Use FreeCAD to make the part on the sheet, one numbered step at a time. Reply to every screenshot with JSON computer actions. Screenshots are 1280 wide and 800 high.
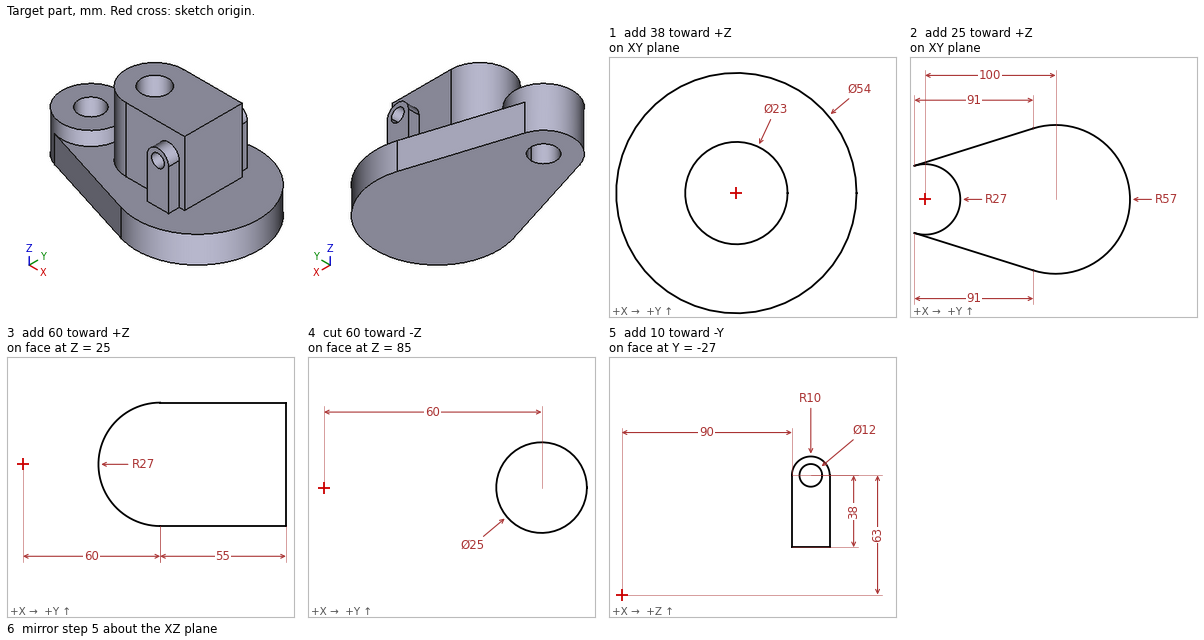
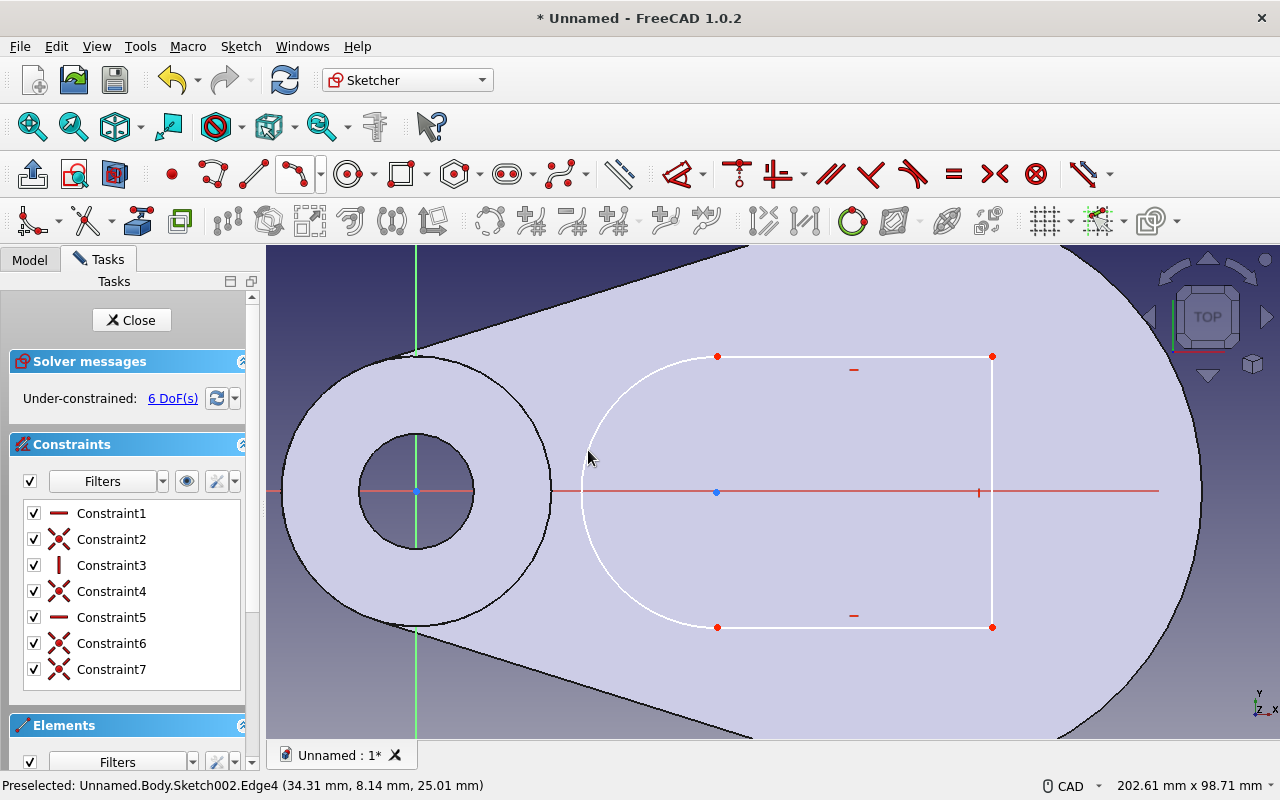
{"action": "left_click", "coordinate": [800, 628]}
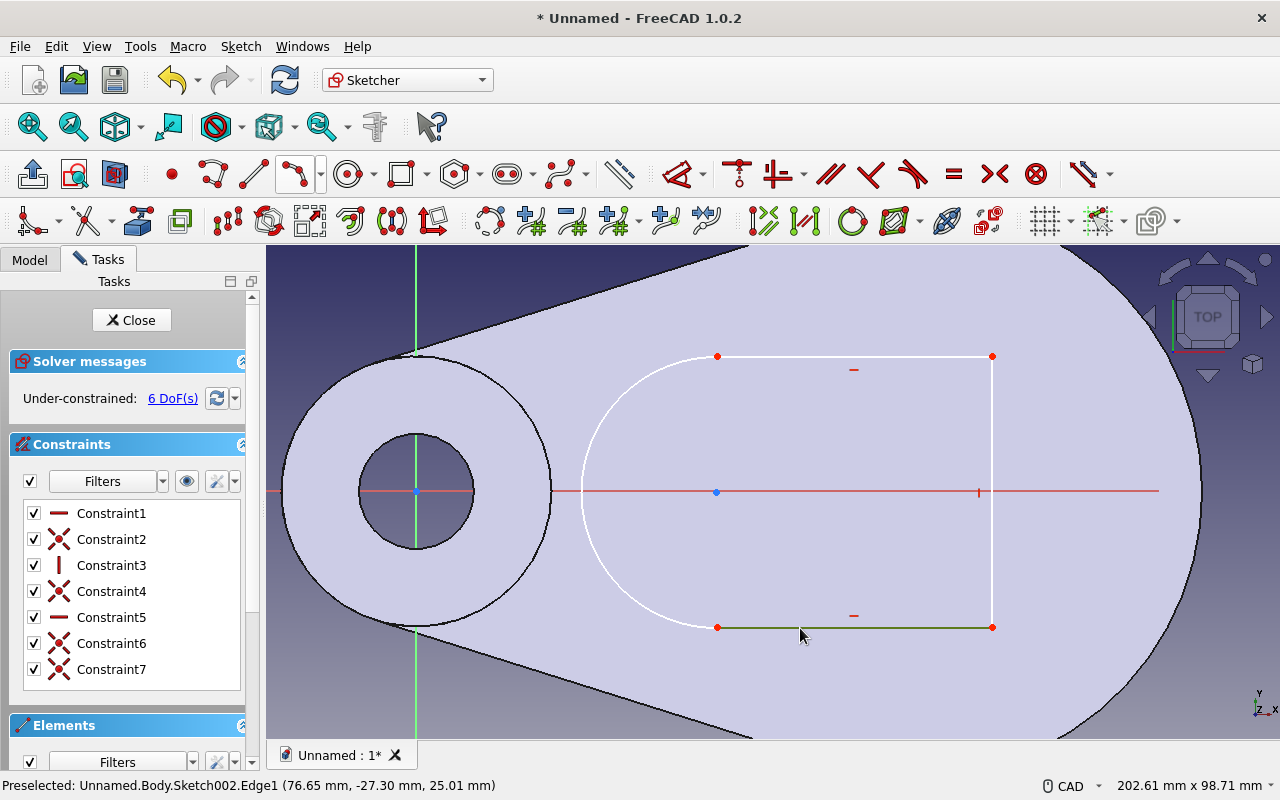
{"action": "left_click", "coordinate": [607, 413]}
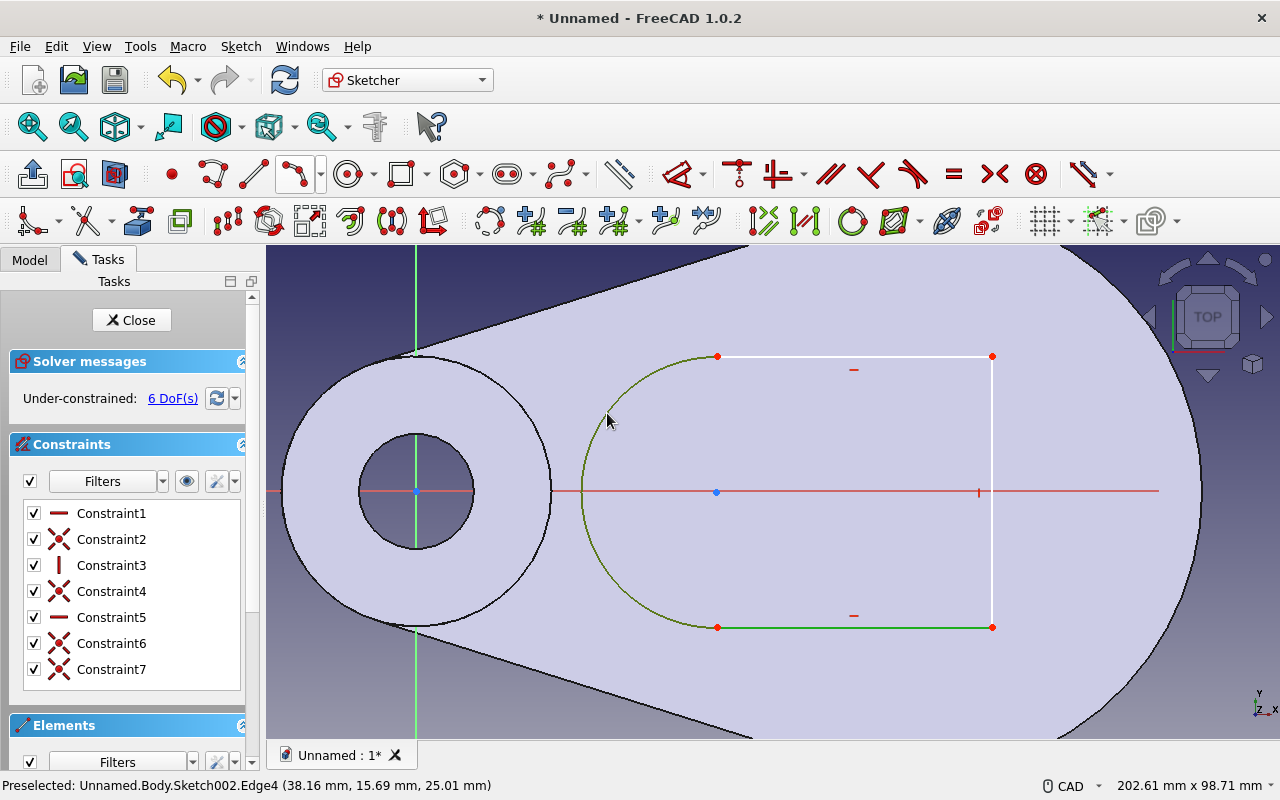
{"action": "key", "text": "t"}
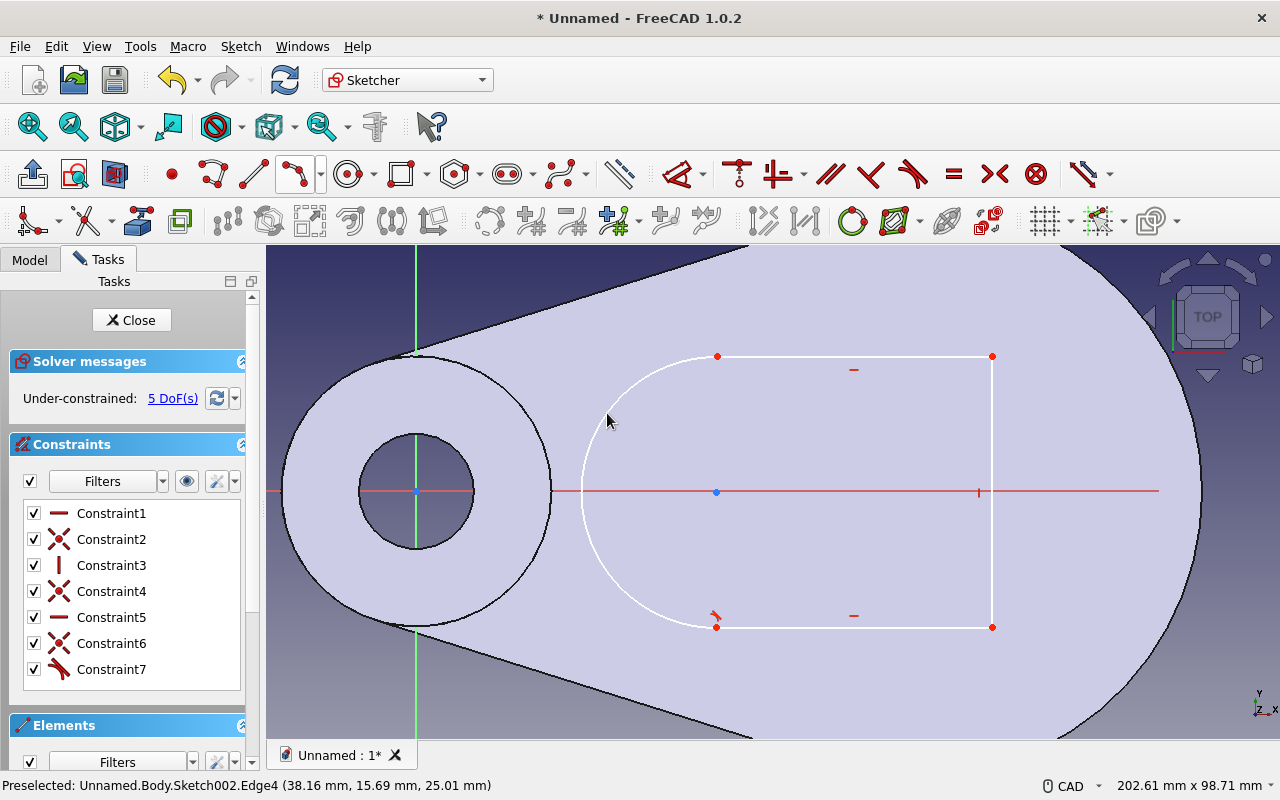
{"action": "left_click", "coordinate": [910, 357]}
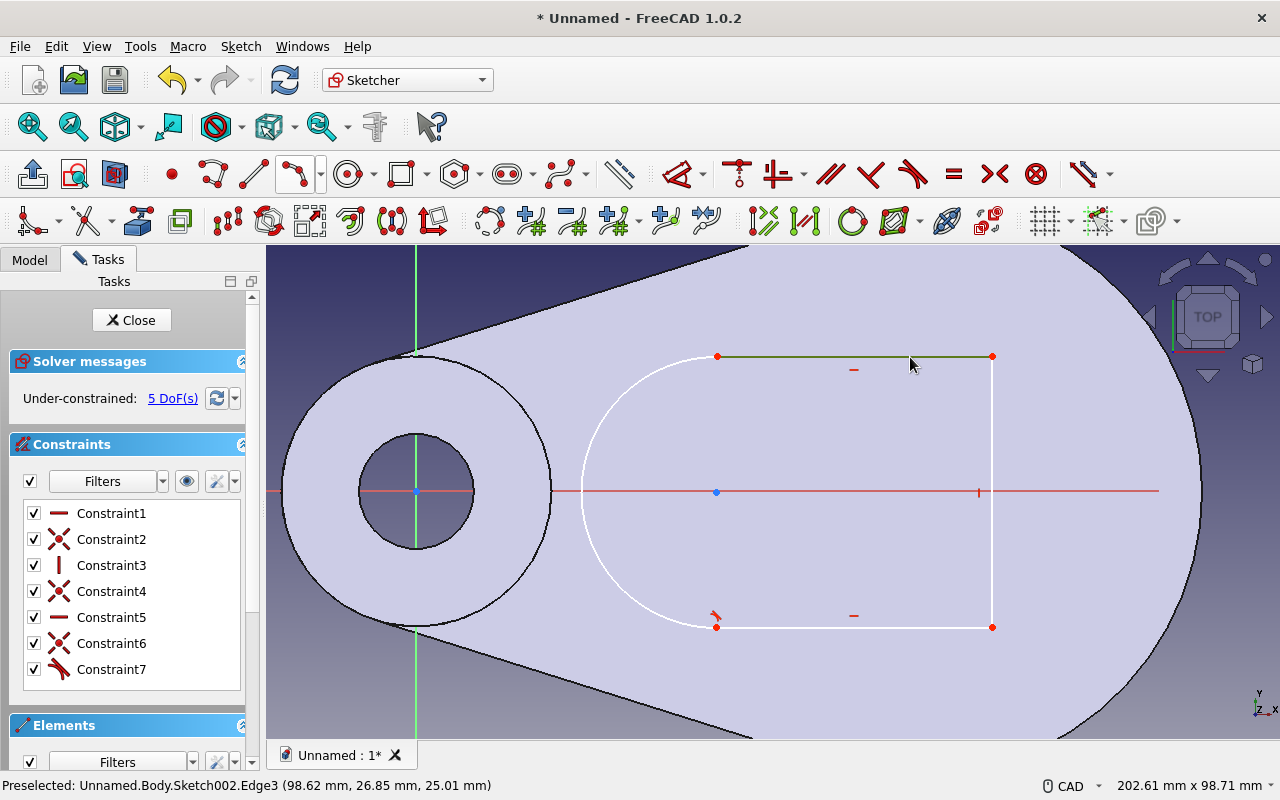
{"action": "left_click", "coordinate": [607, 413]}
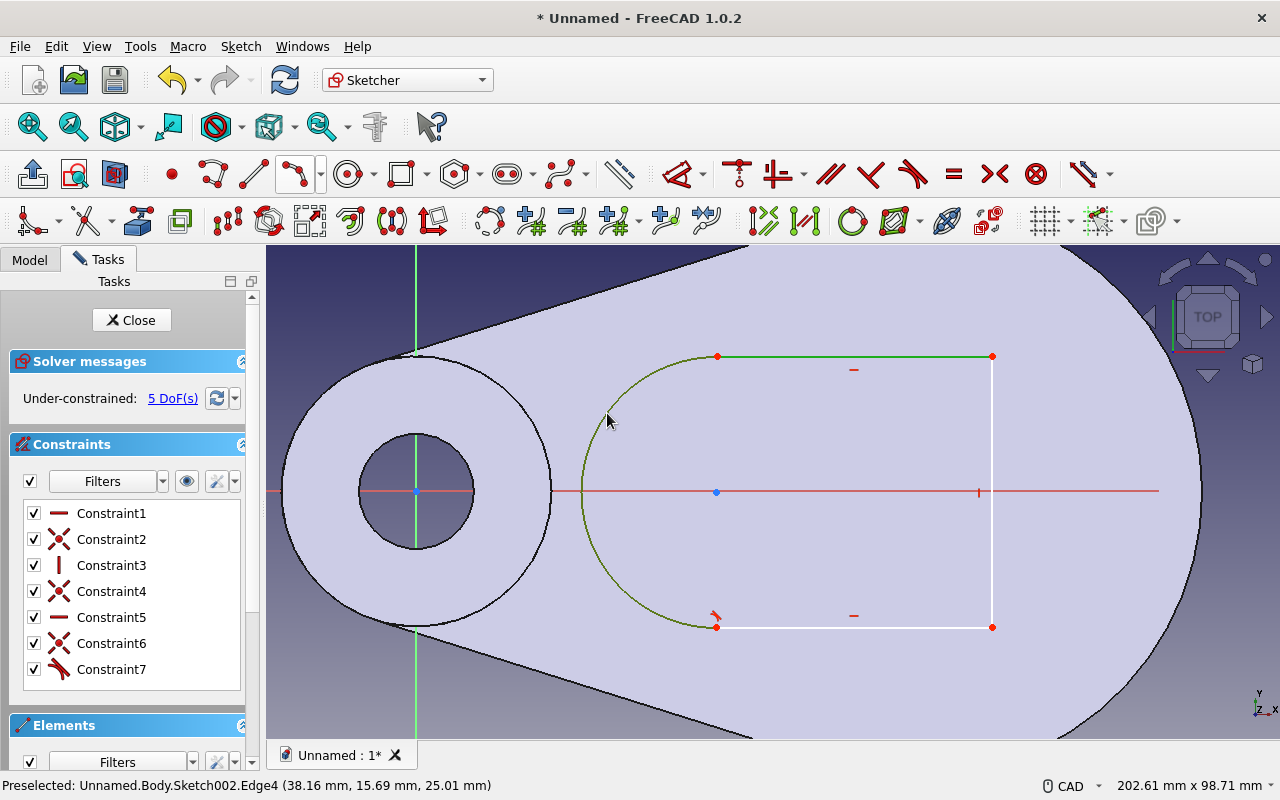
{"action": "key", "text": "t"}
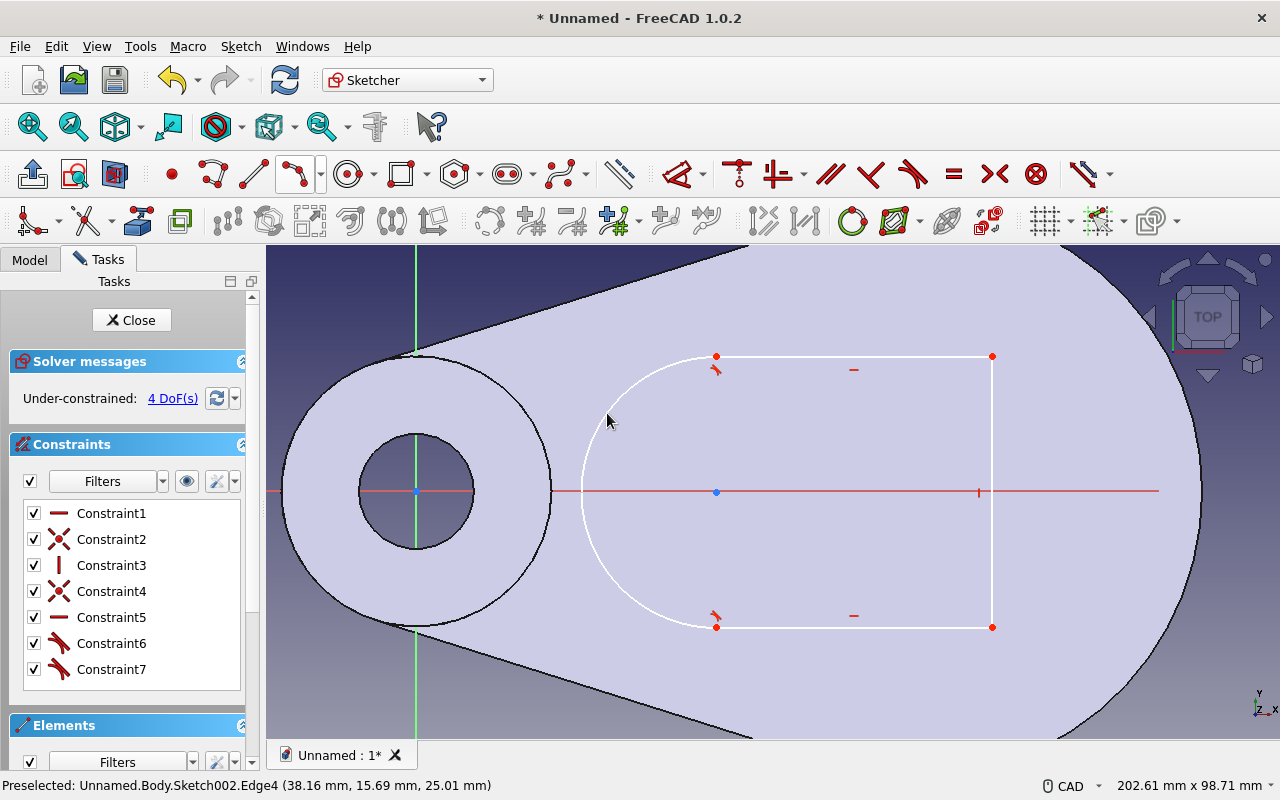
{"action": "left_click", "coordinate": [717, 492]}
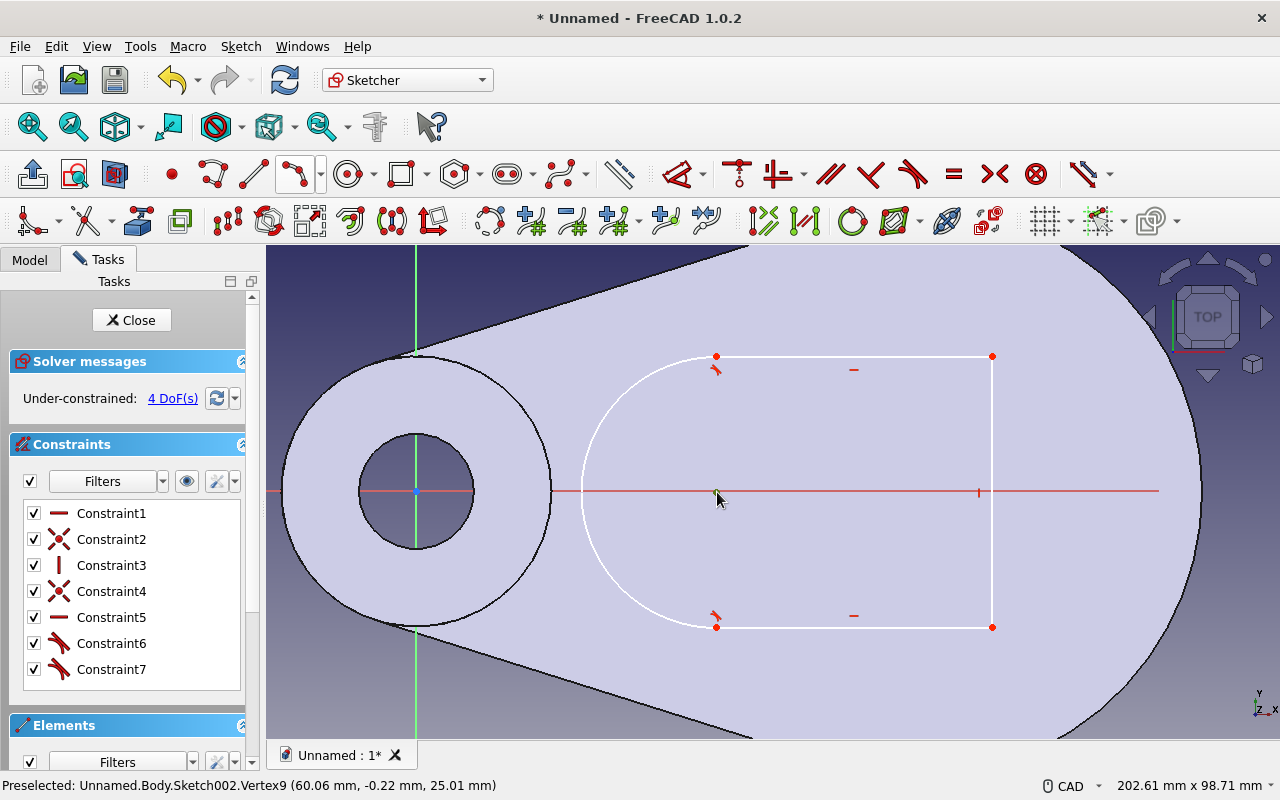
{"action": "left_click", "coordinate": [353, 491]}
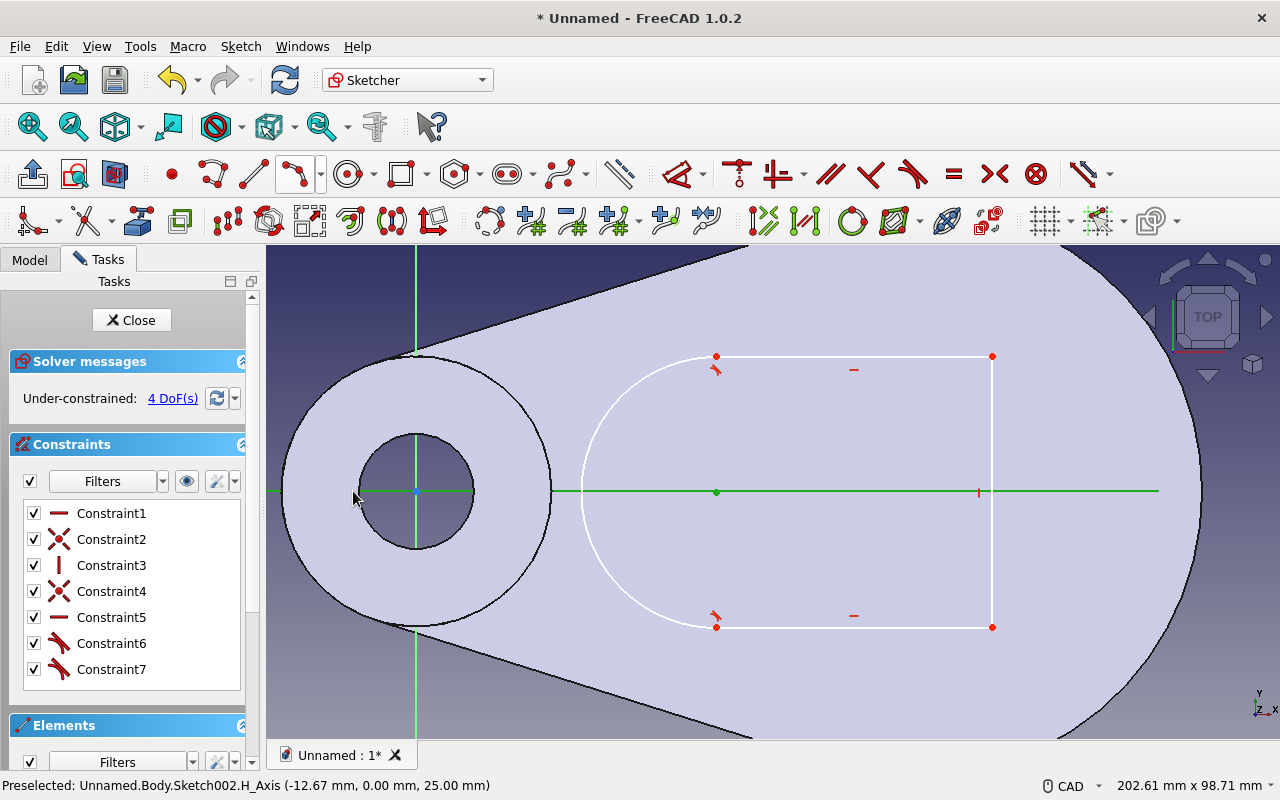
{"action": "left_click", "coordinate": [737, 174]}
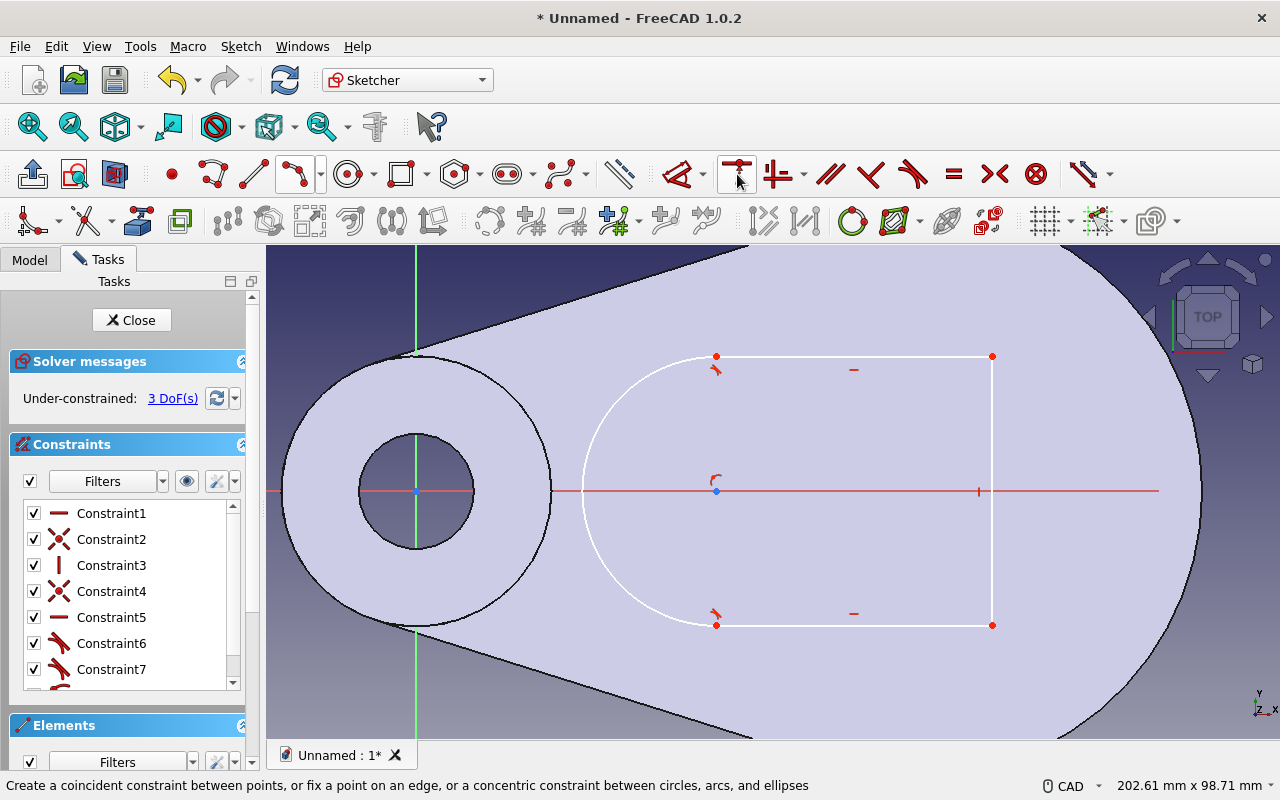
{"action": "key", "text": "d"}